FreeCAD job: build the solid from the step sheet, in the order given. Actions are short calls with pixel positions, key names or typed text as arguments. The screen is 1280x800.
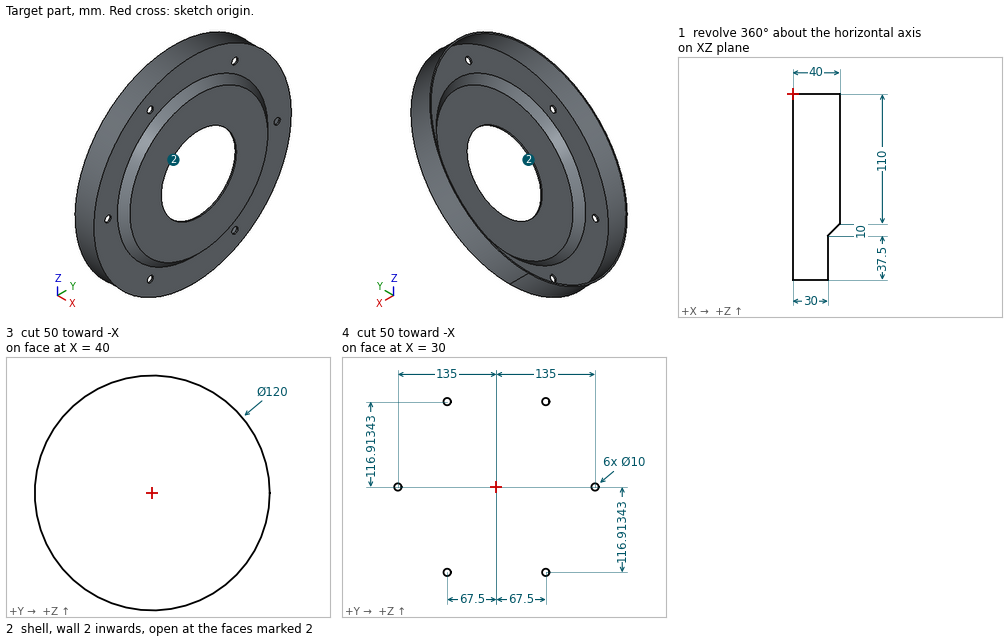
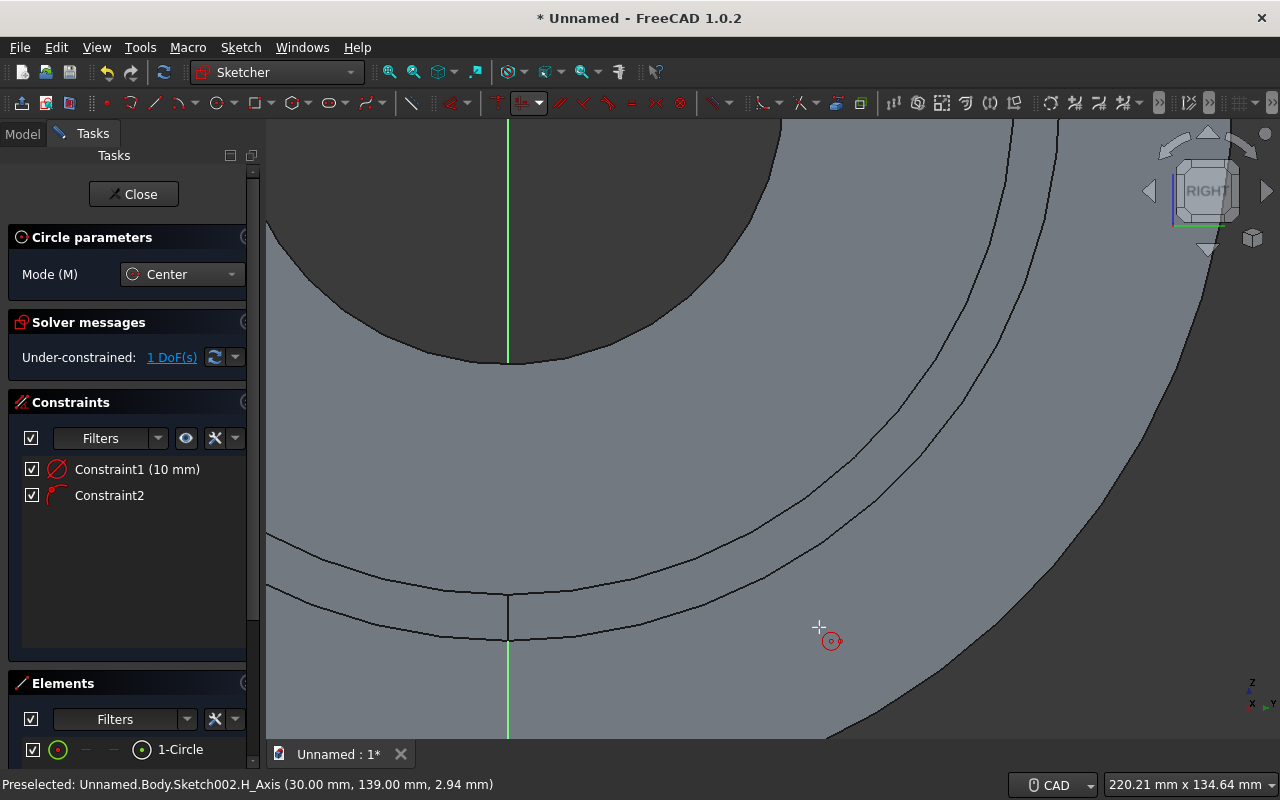
click(819, 627)
move(835, 610)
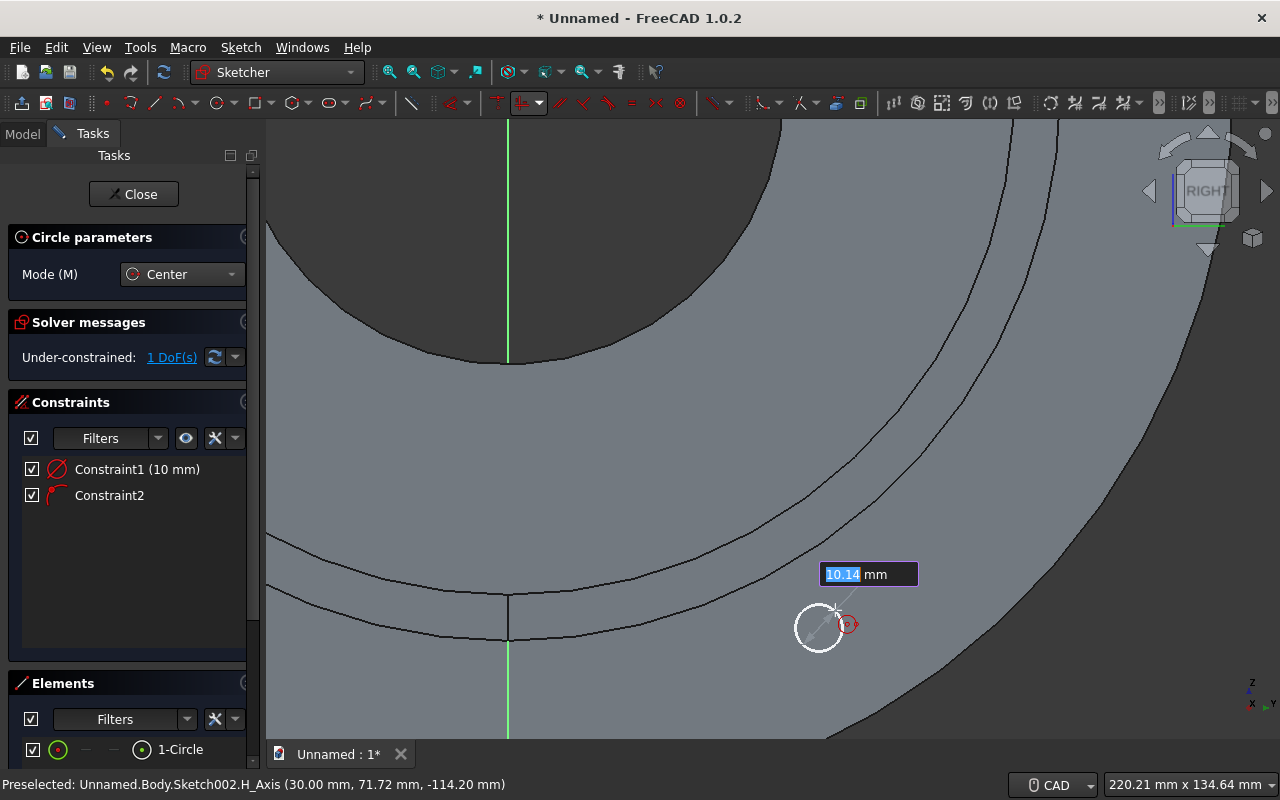
text(10)
key(Return)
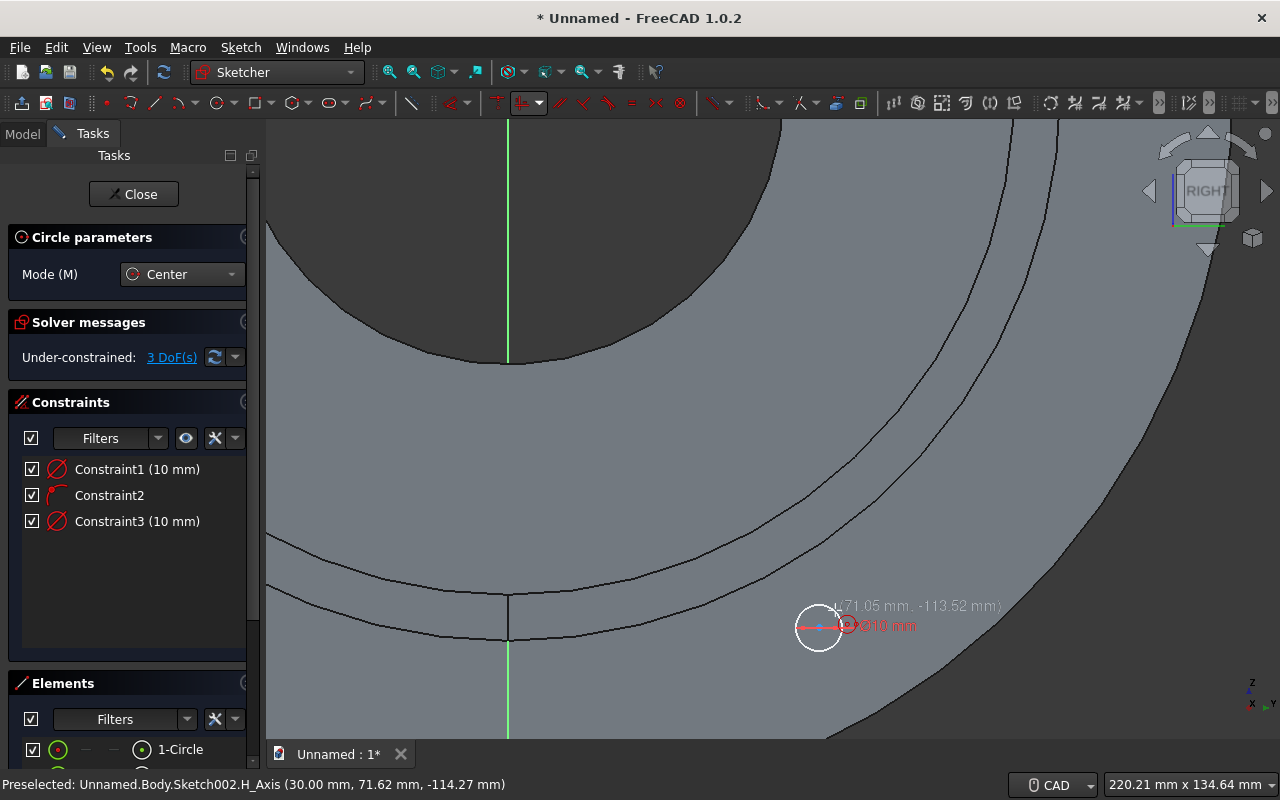
scroll(819, 627, down, 5)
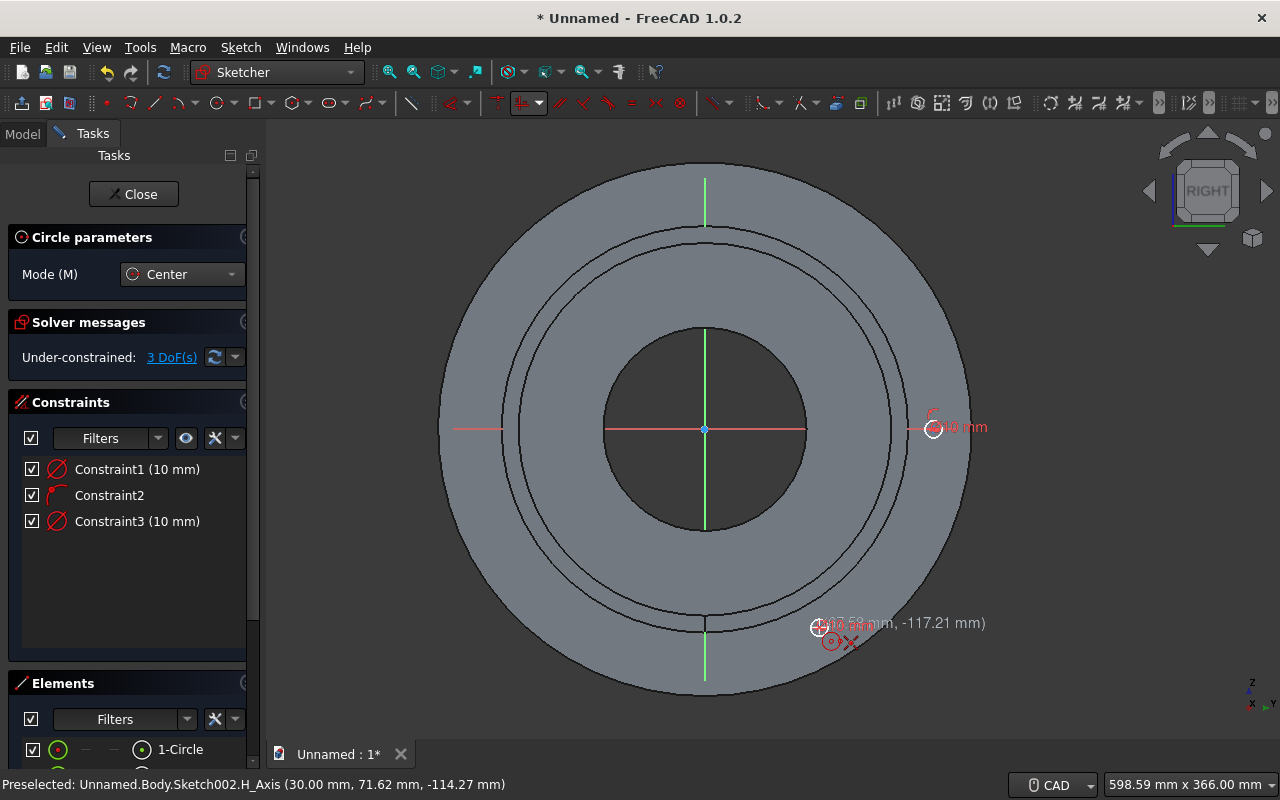
scroll(591, 627, up, 5)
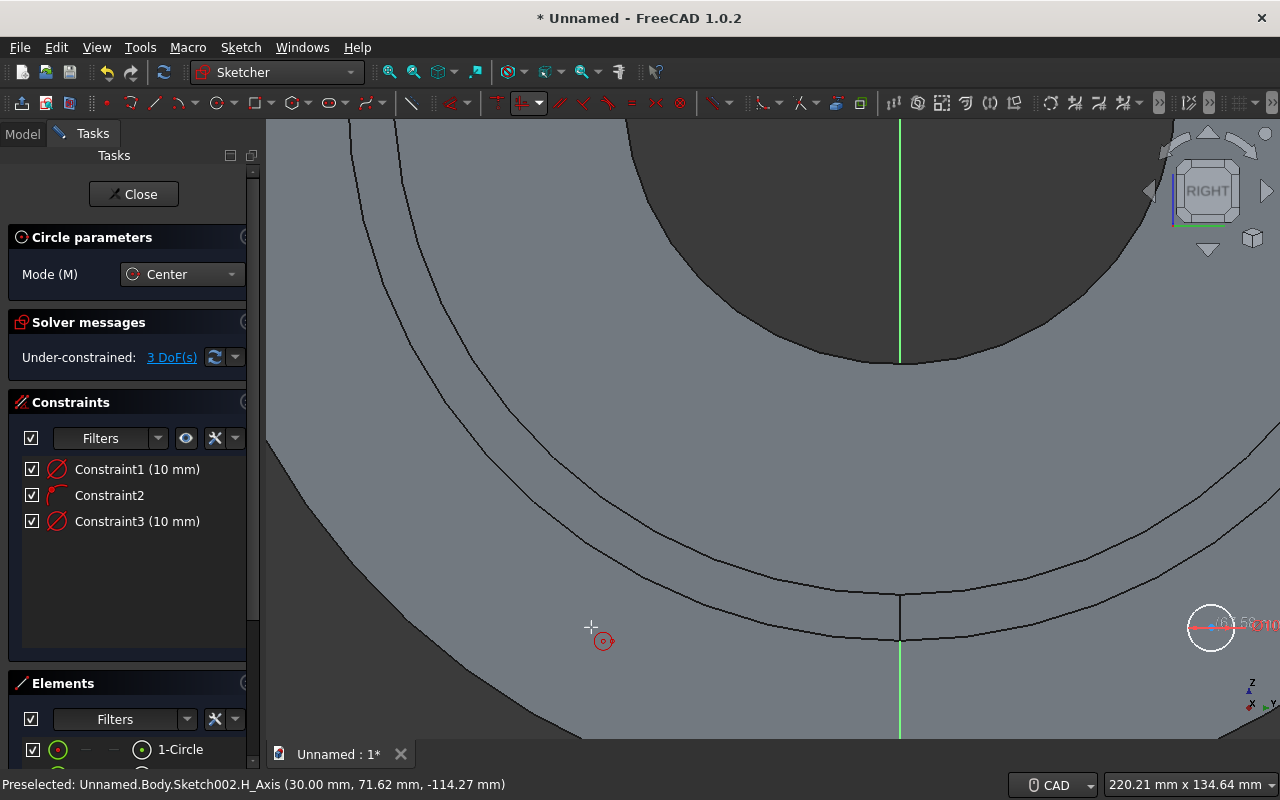
click(589, 627)
move(605, 610)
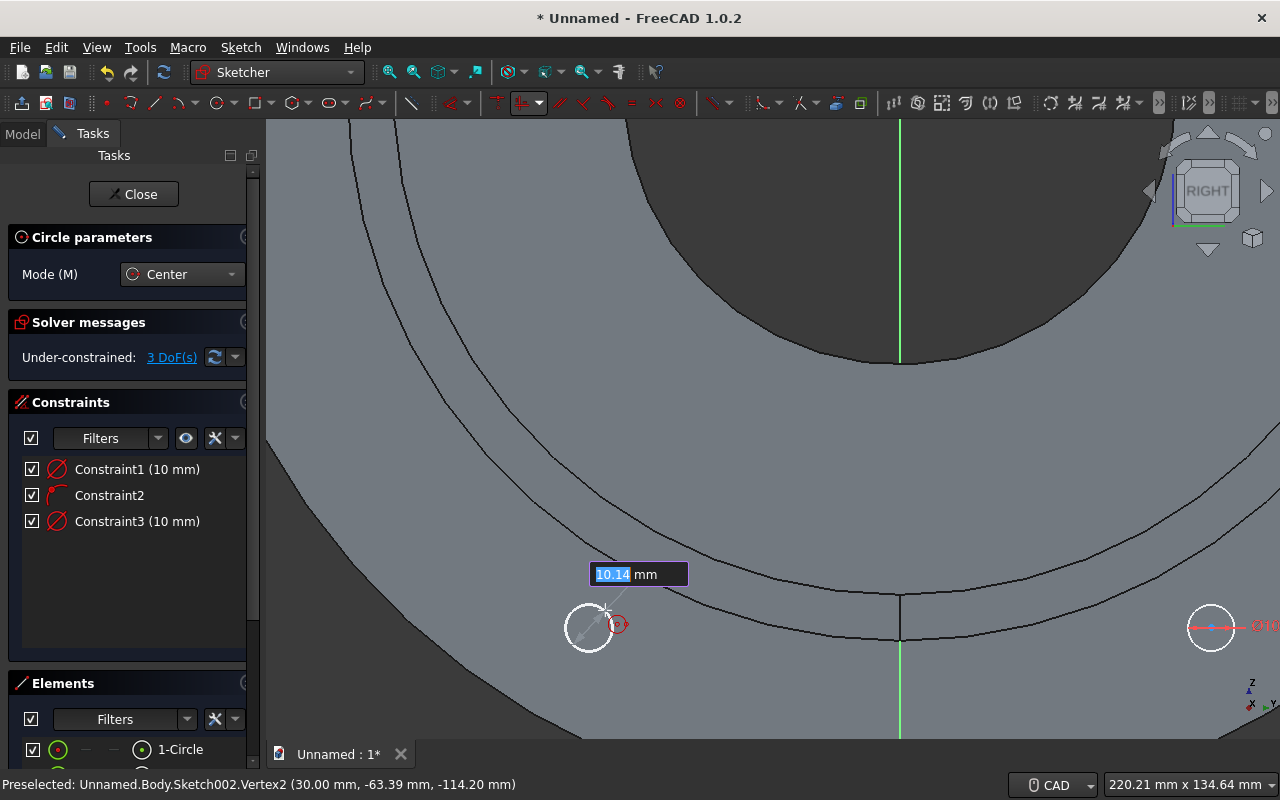
text(10)
key(Return)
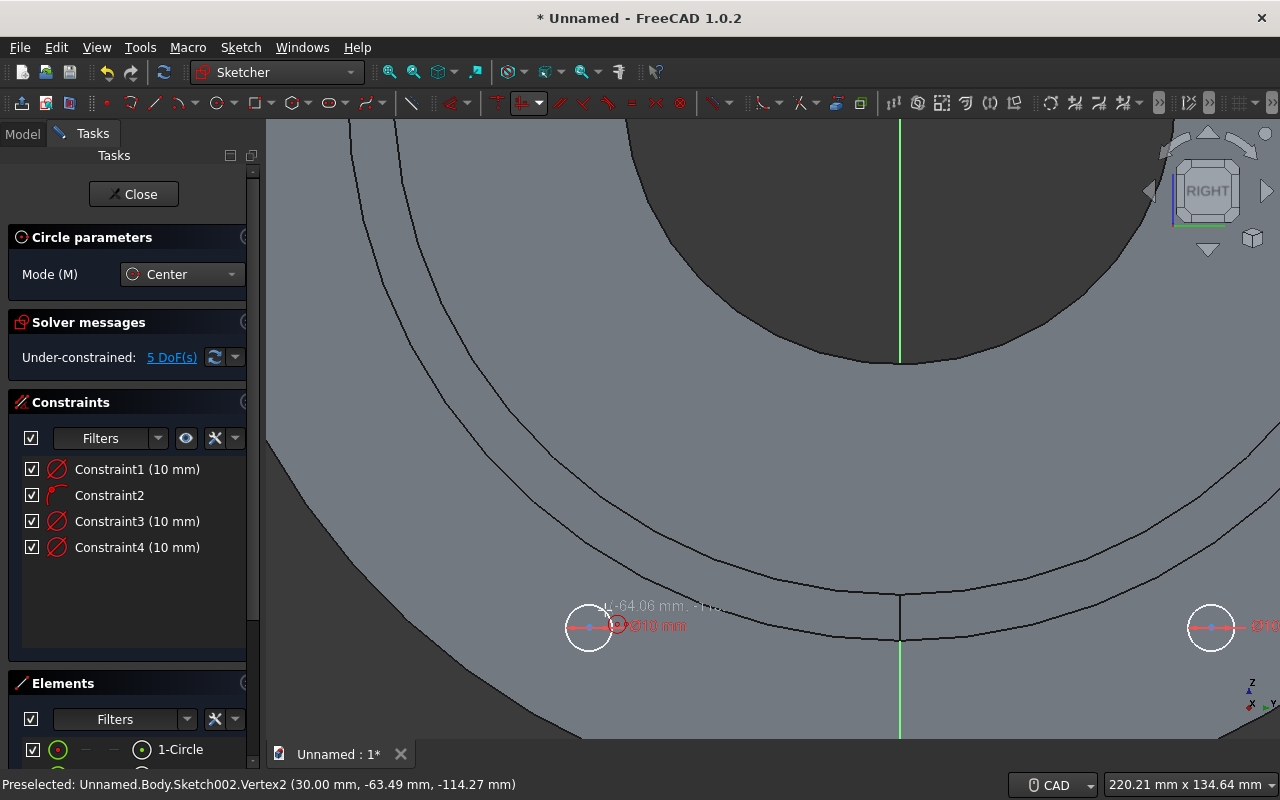
scroll(591, 627, down, 5)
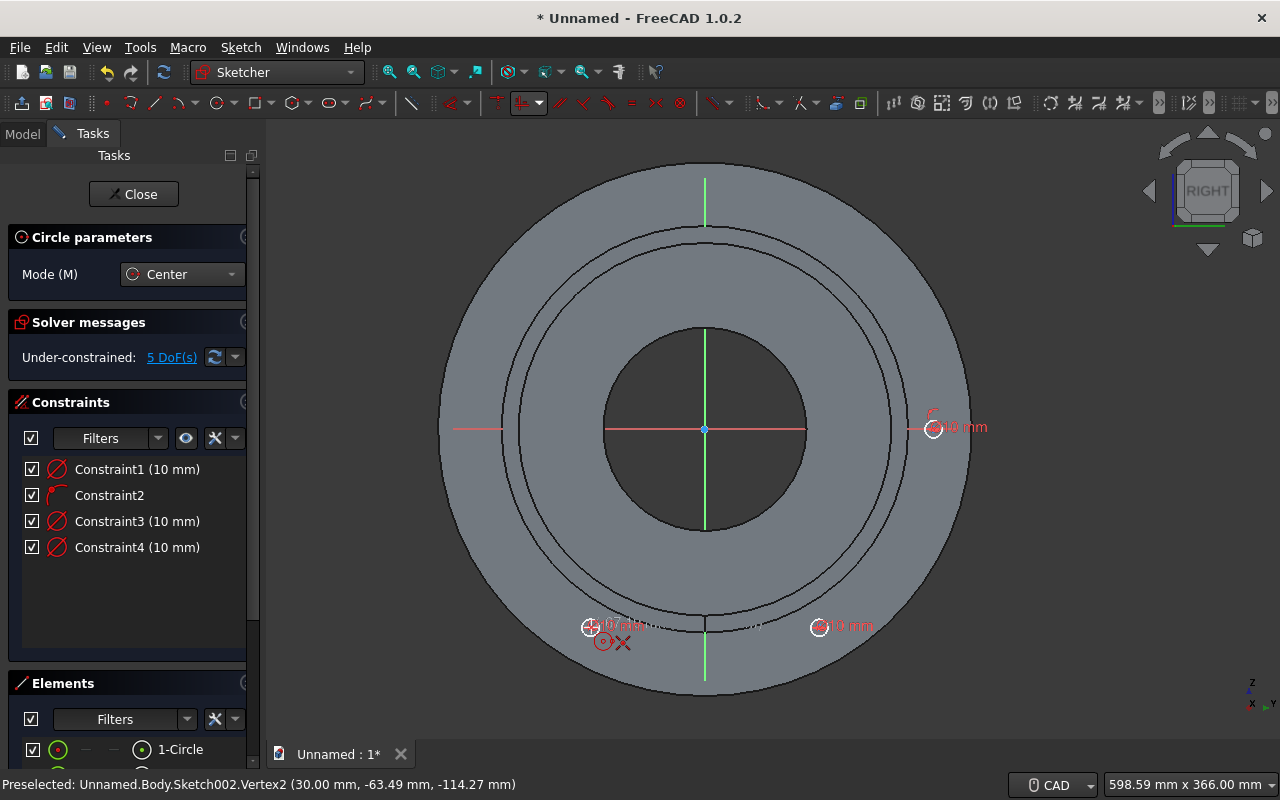
scroll(476, 429, up, 5)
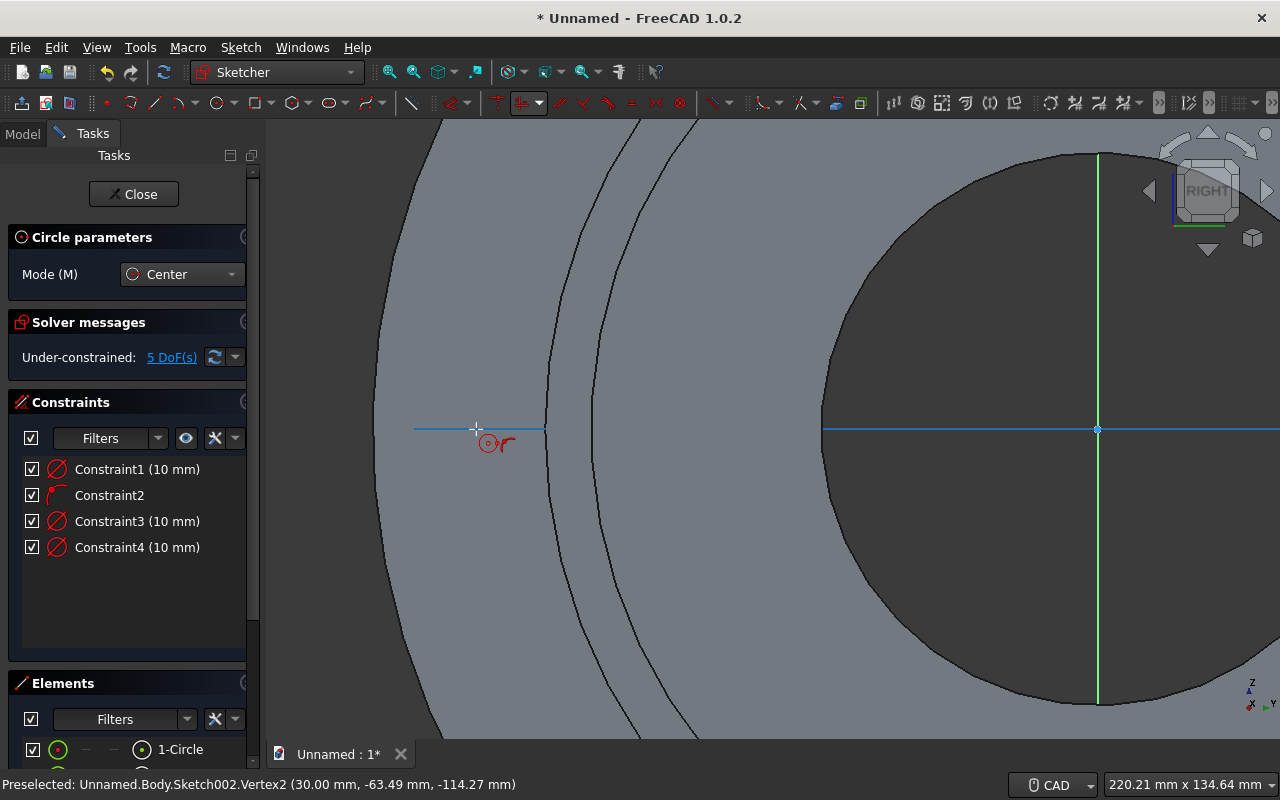
click(476, 429)
move(492, 413)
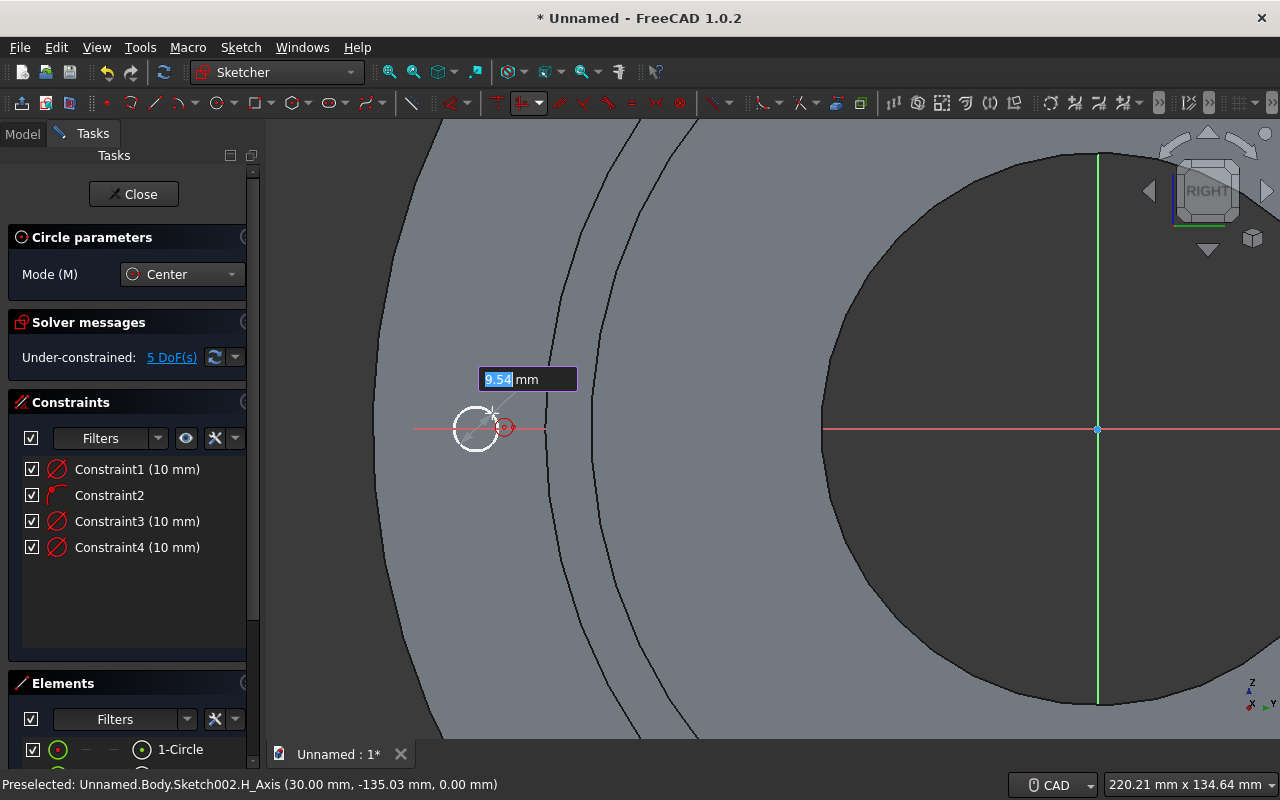
text(10)
key(Return)